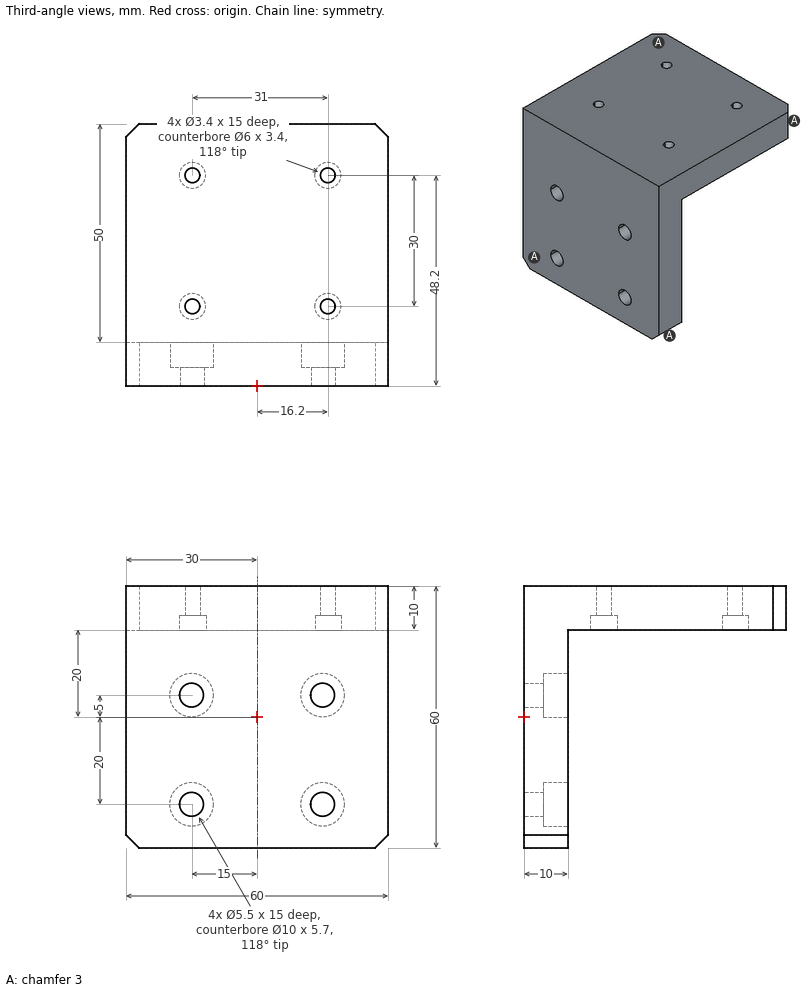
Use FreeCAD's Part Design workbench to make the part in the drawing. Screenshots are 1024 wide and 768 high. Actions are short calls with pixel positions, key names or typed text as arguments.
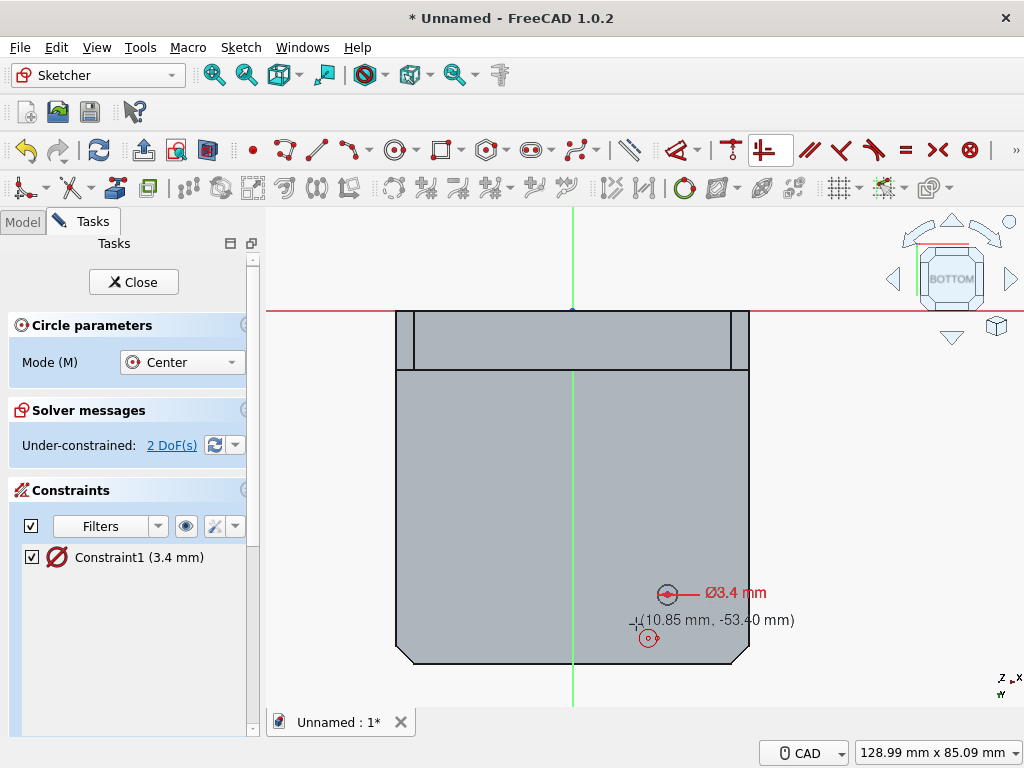
scroll(486, 594, up, 5)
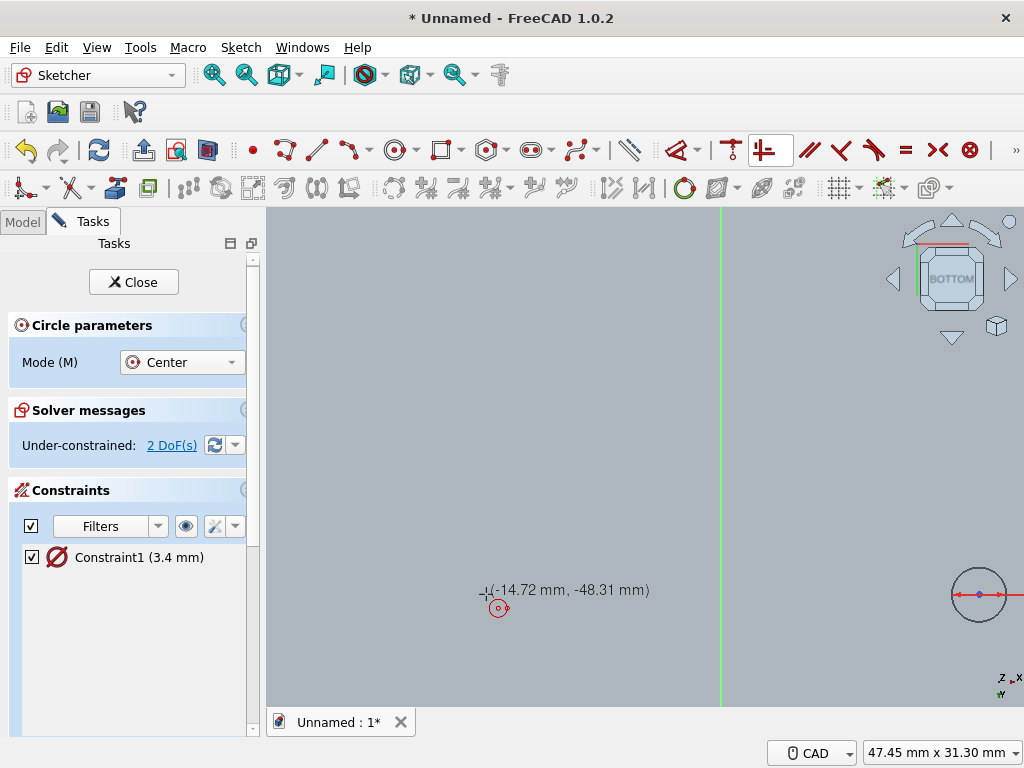
click(484, 594)
move(504, 574)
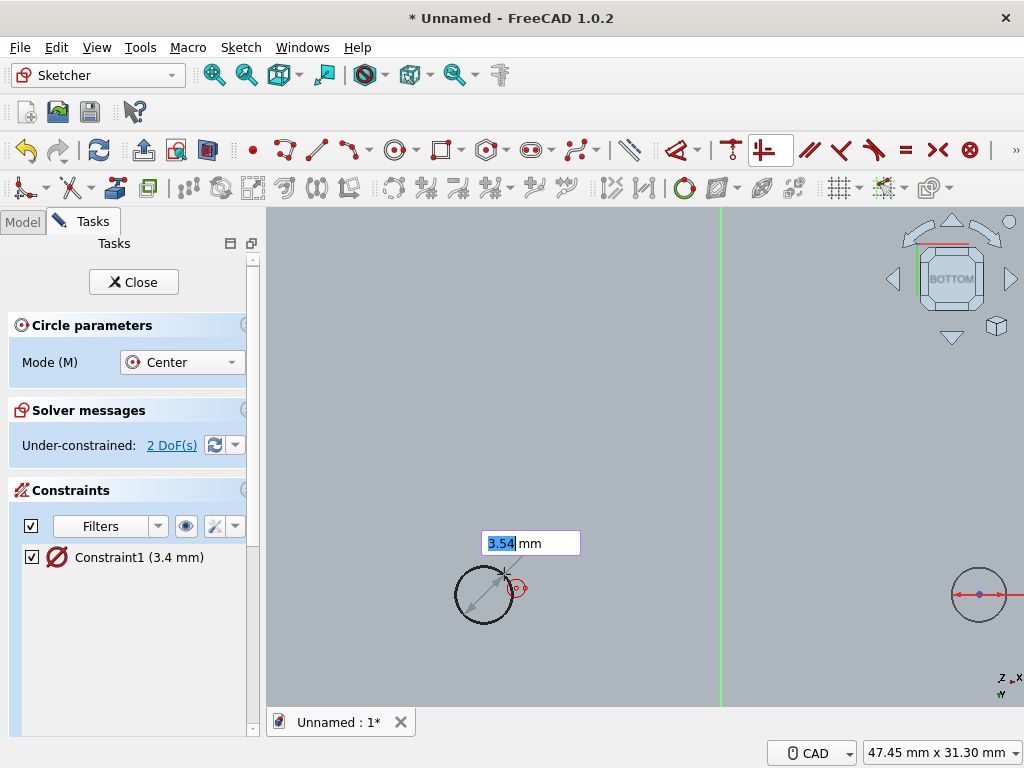
text(3.4)
key(Return)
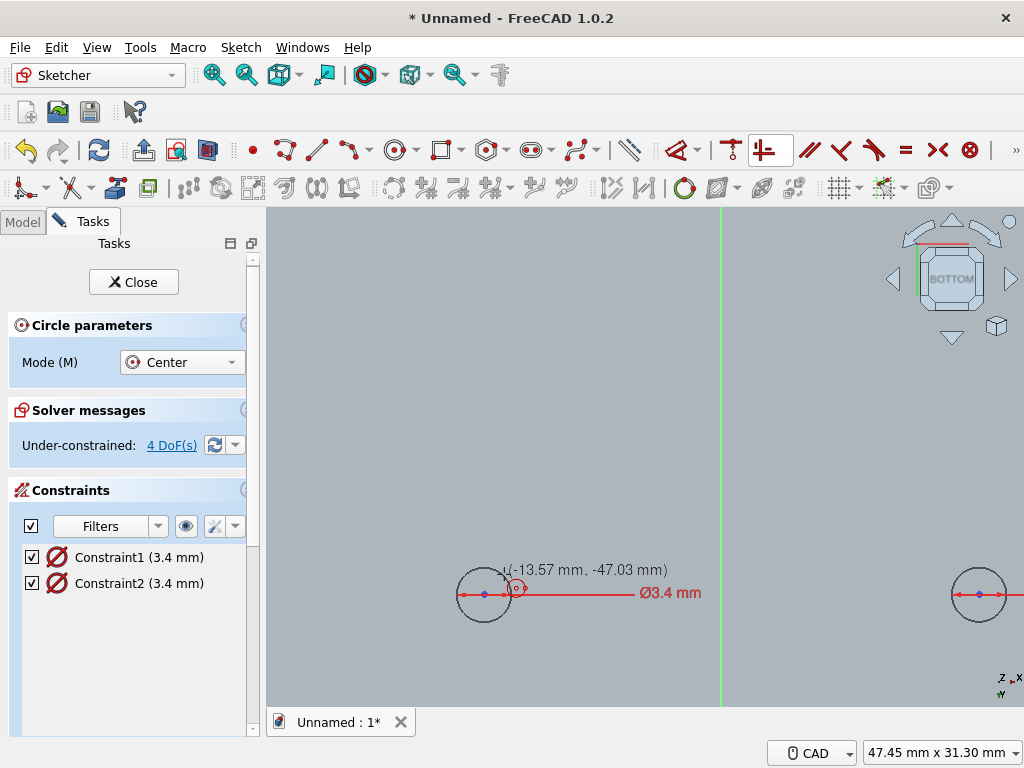
scroll(486, 594, down, 5)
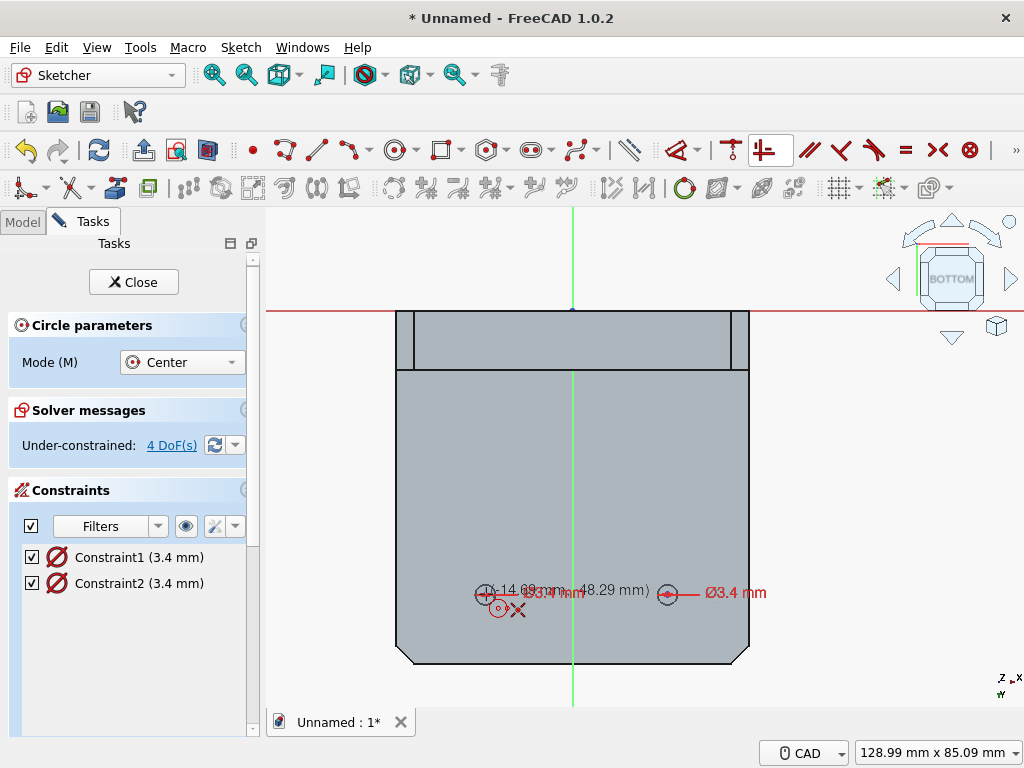
scroll(668, 418, up, 5)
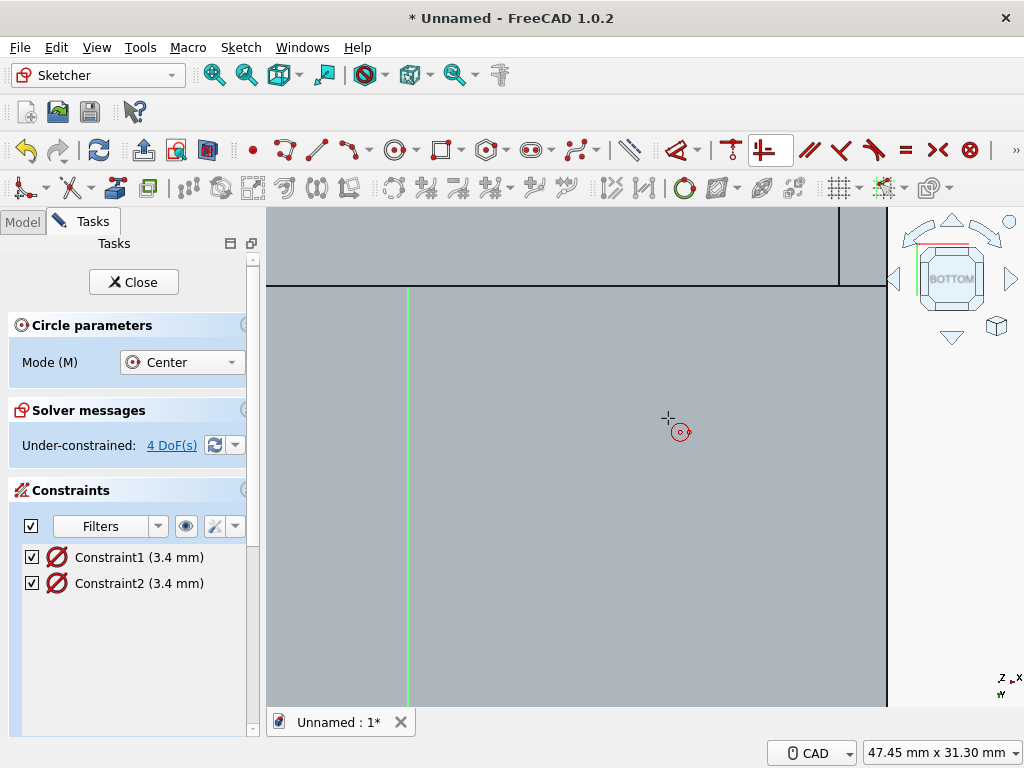
click(666, 417)
move(686, 398)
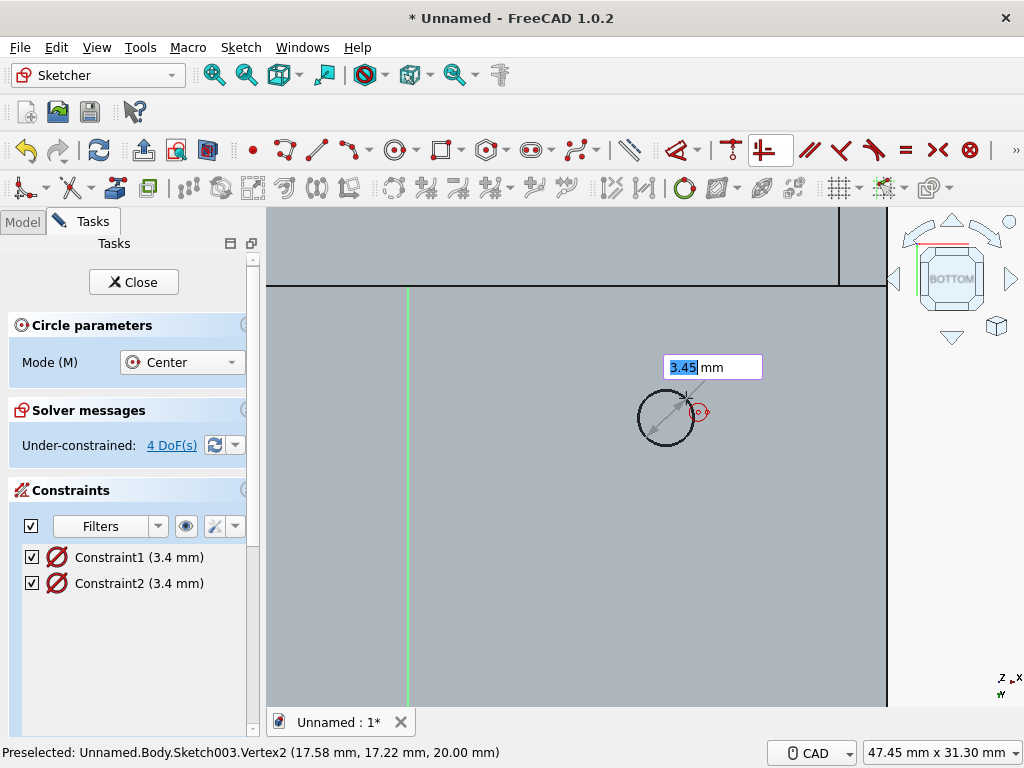
text(3.4)
key(Return)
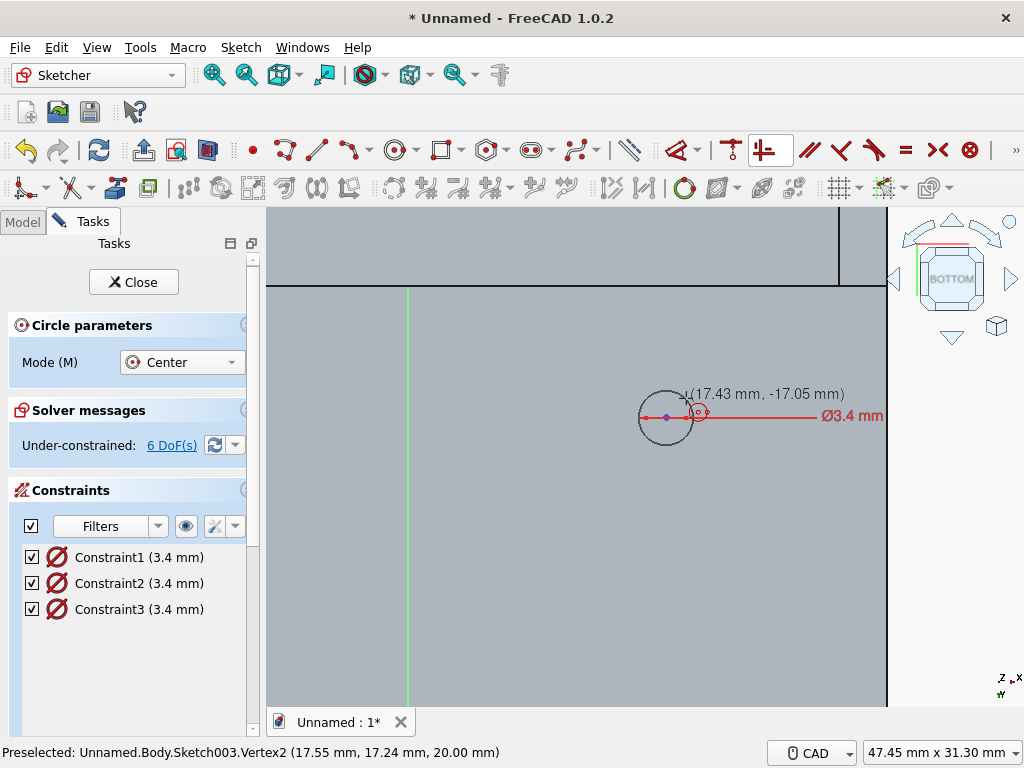
scroll(668, 417, down, 5)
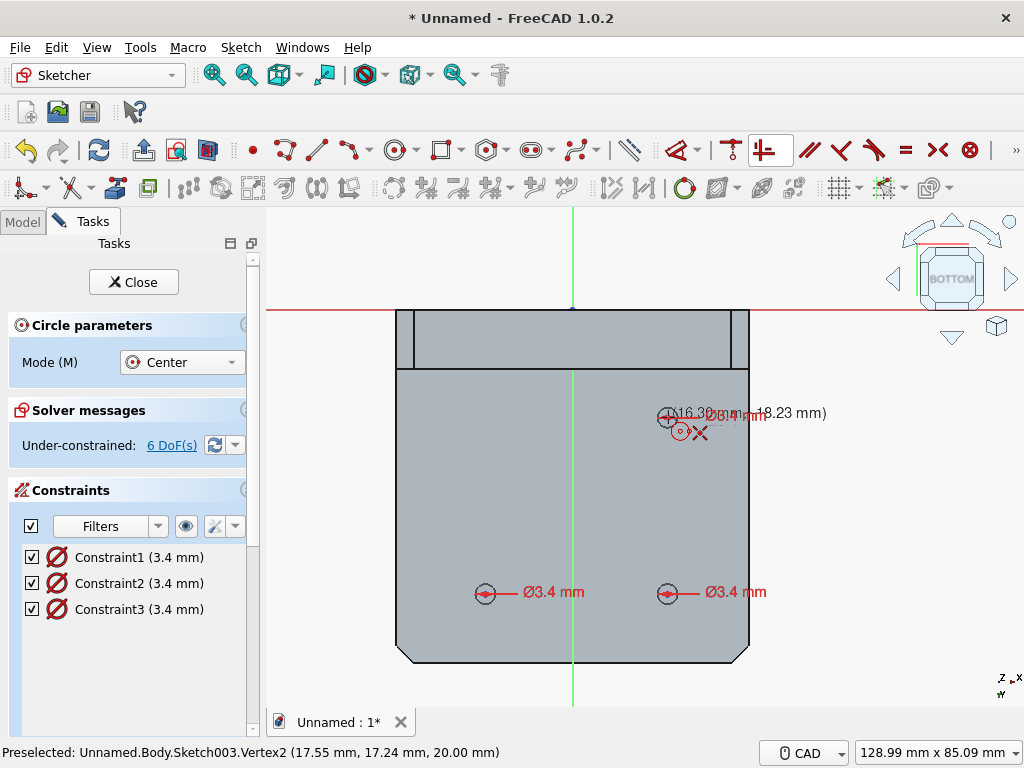
scroll(486, 417, up, 5)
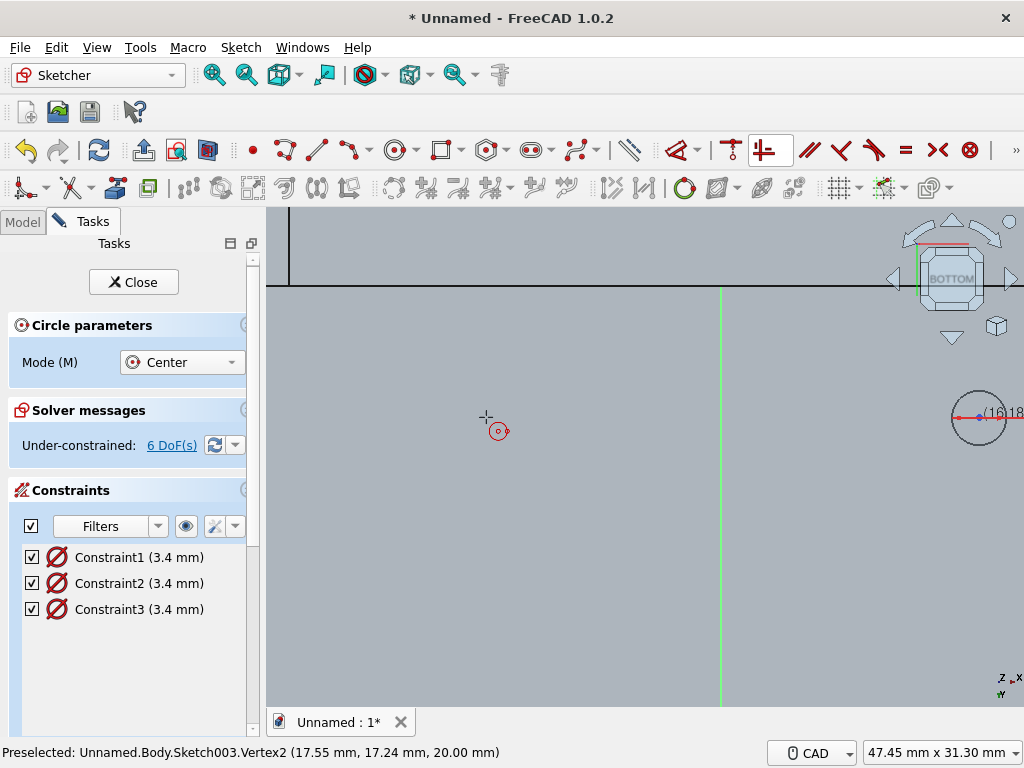
click(484, 417)
move(504, 398)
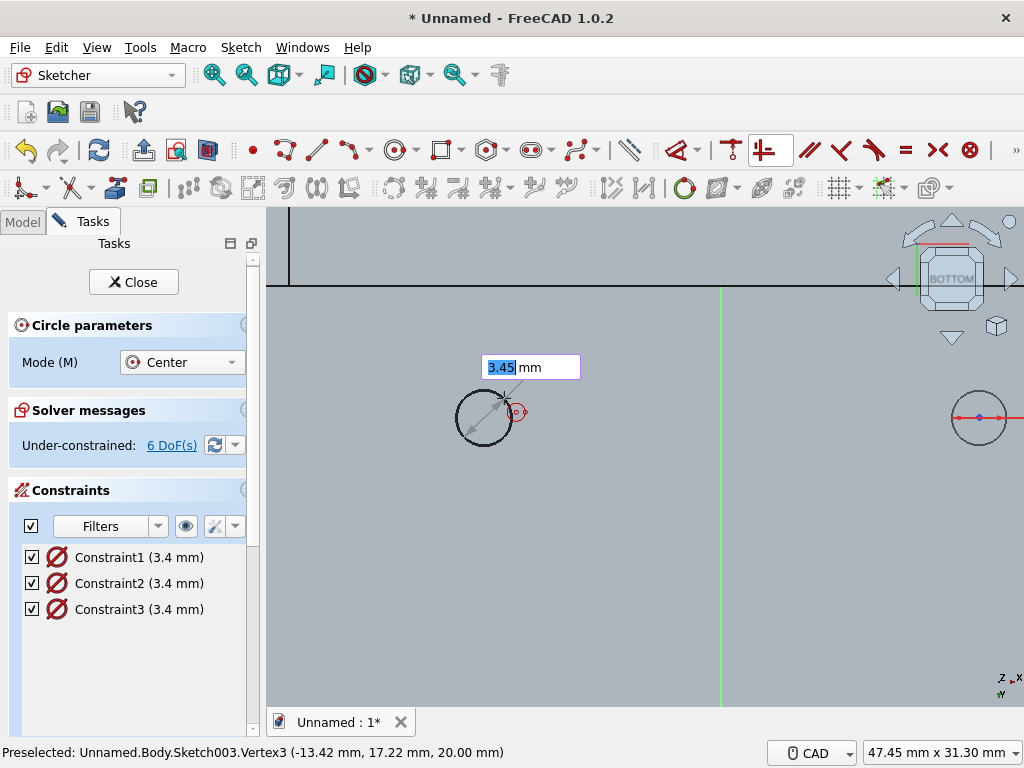
text(3.4)
key(Return)
key(Escape)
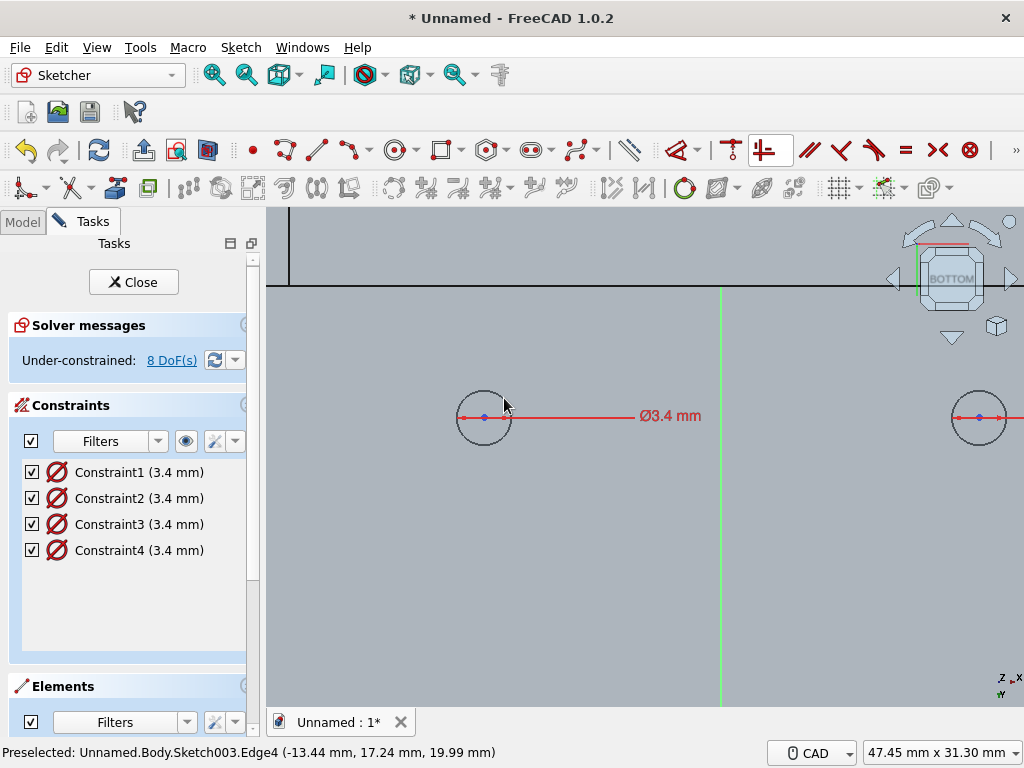
key(d)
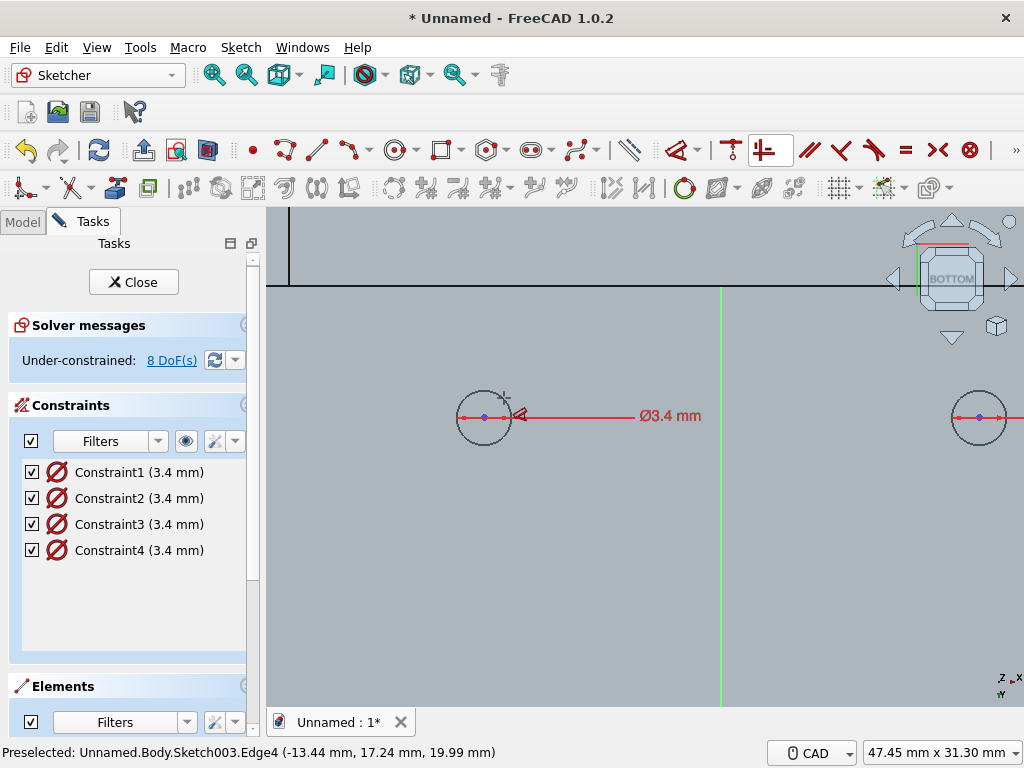
scroll(486, 417, down, 5)